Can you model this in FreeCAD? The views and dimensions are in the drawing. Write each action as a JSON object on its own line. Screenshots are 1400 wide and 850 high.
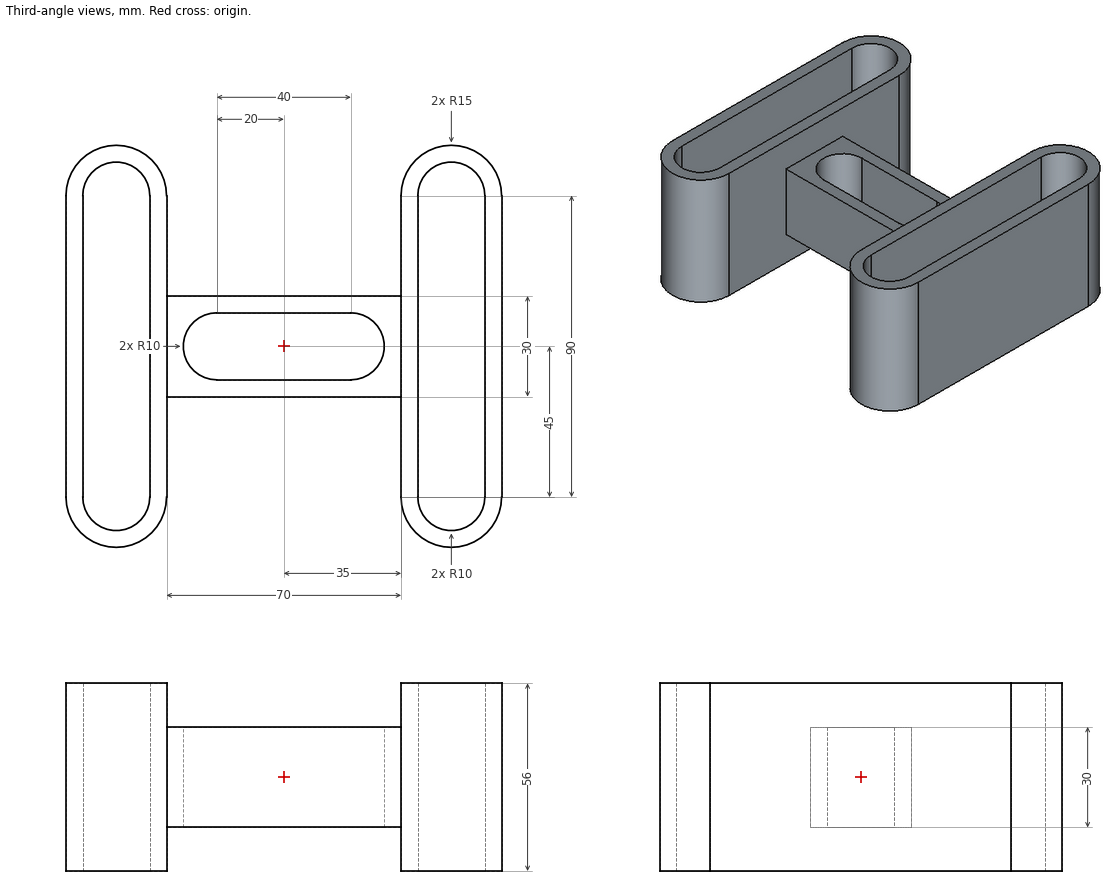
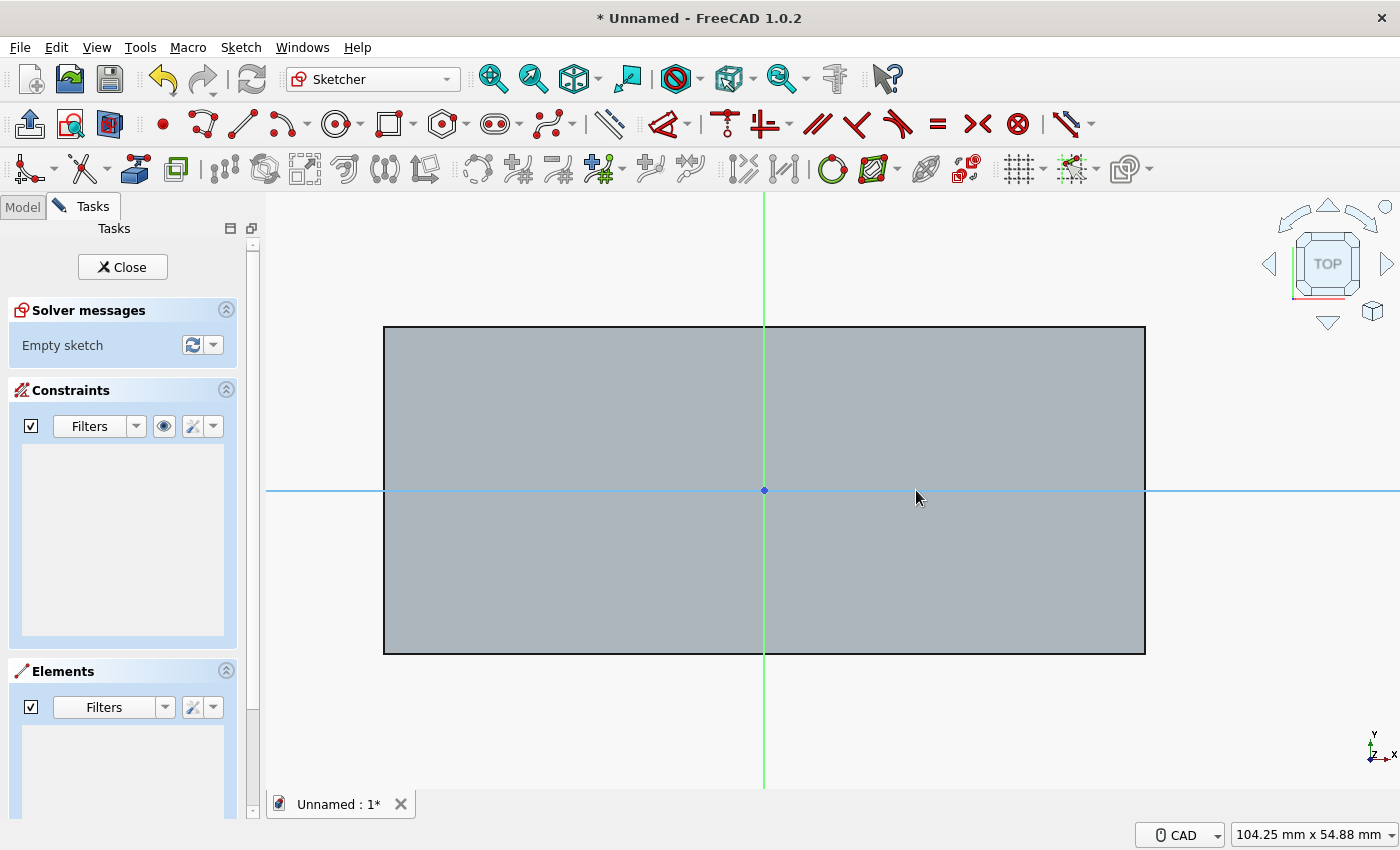
{"action": "left_click", "coordinate": [496, 124]}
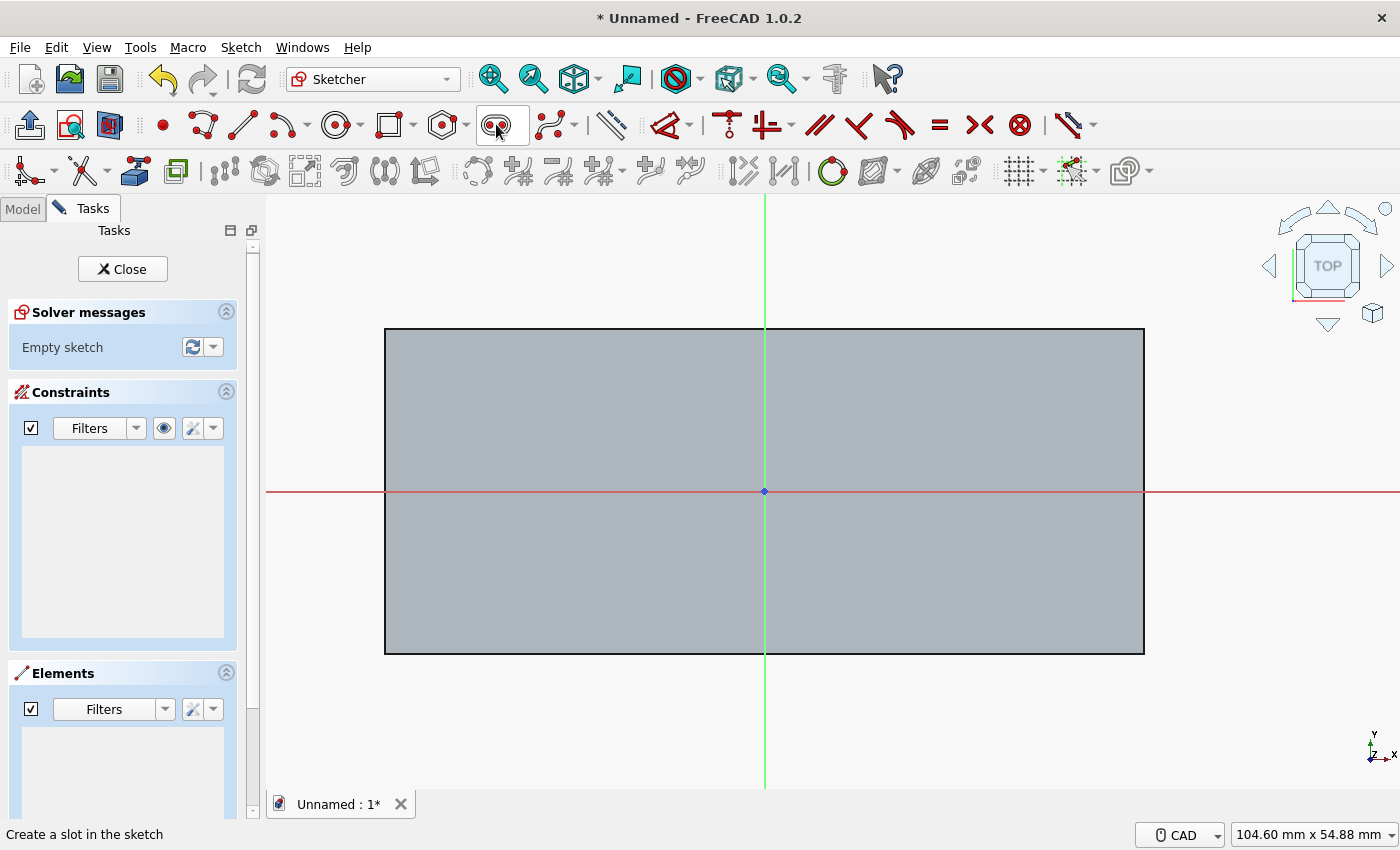
{"action": "left_click", "coordinate": [548, 492]}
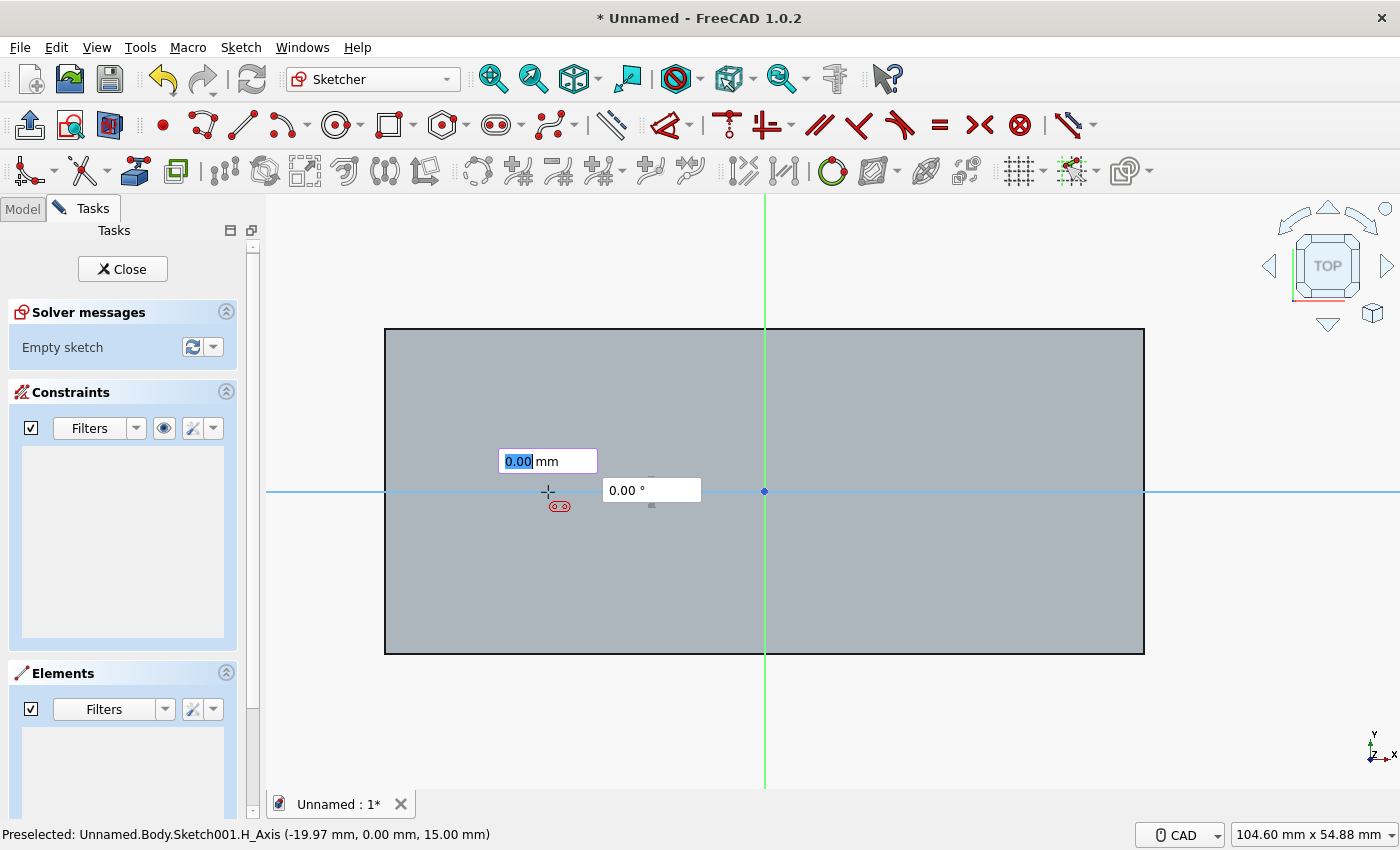
{"action": "left_click", "coordinate": [981, 482]}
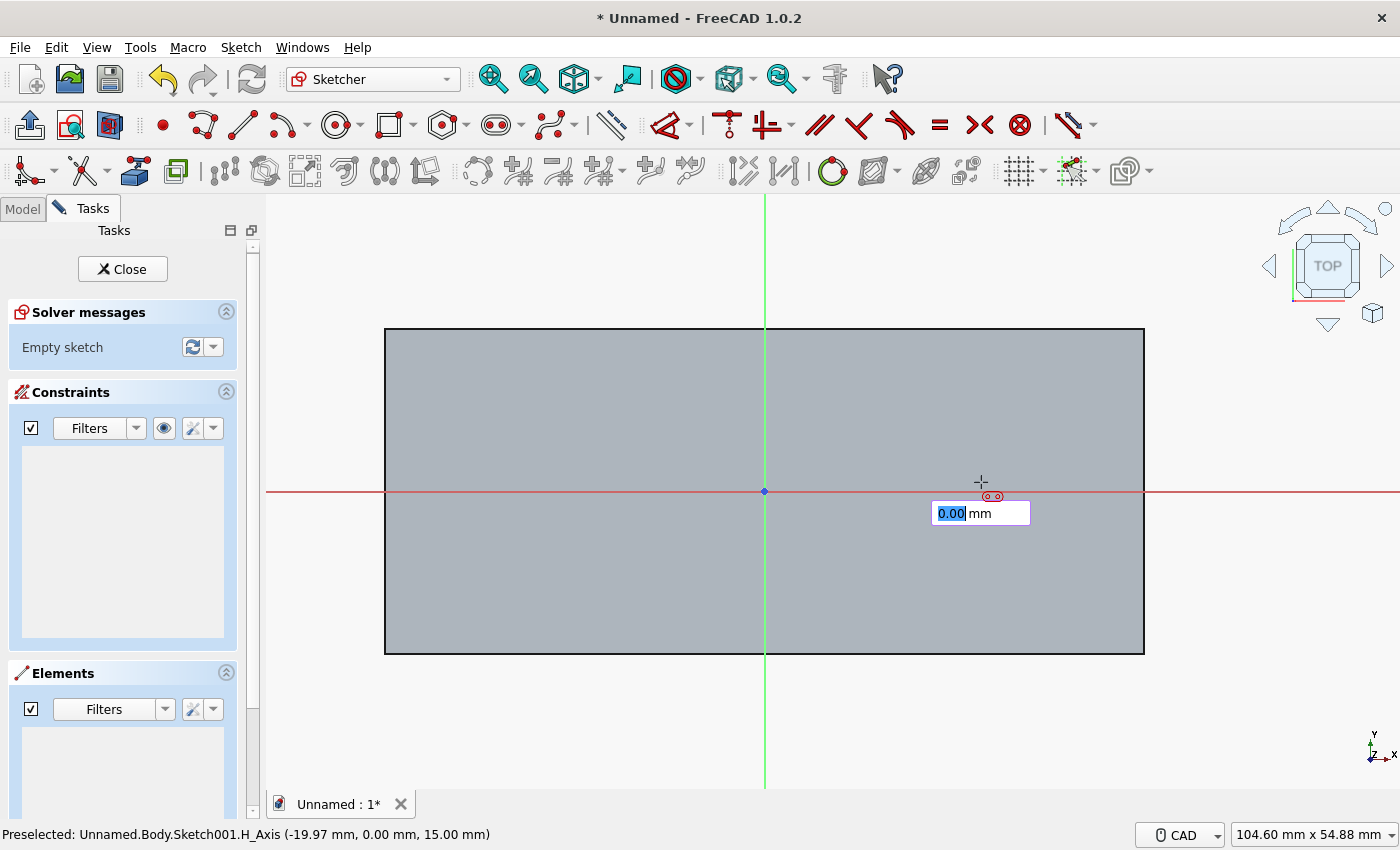
{"action": "left_click", "coordinate": [830, 383]}
{"action": "key", "text": "Escape"}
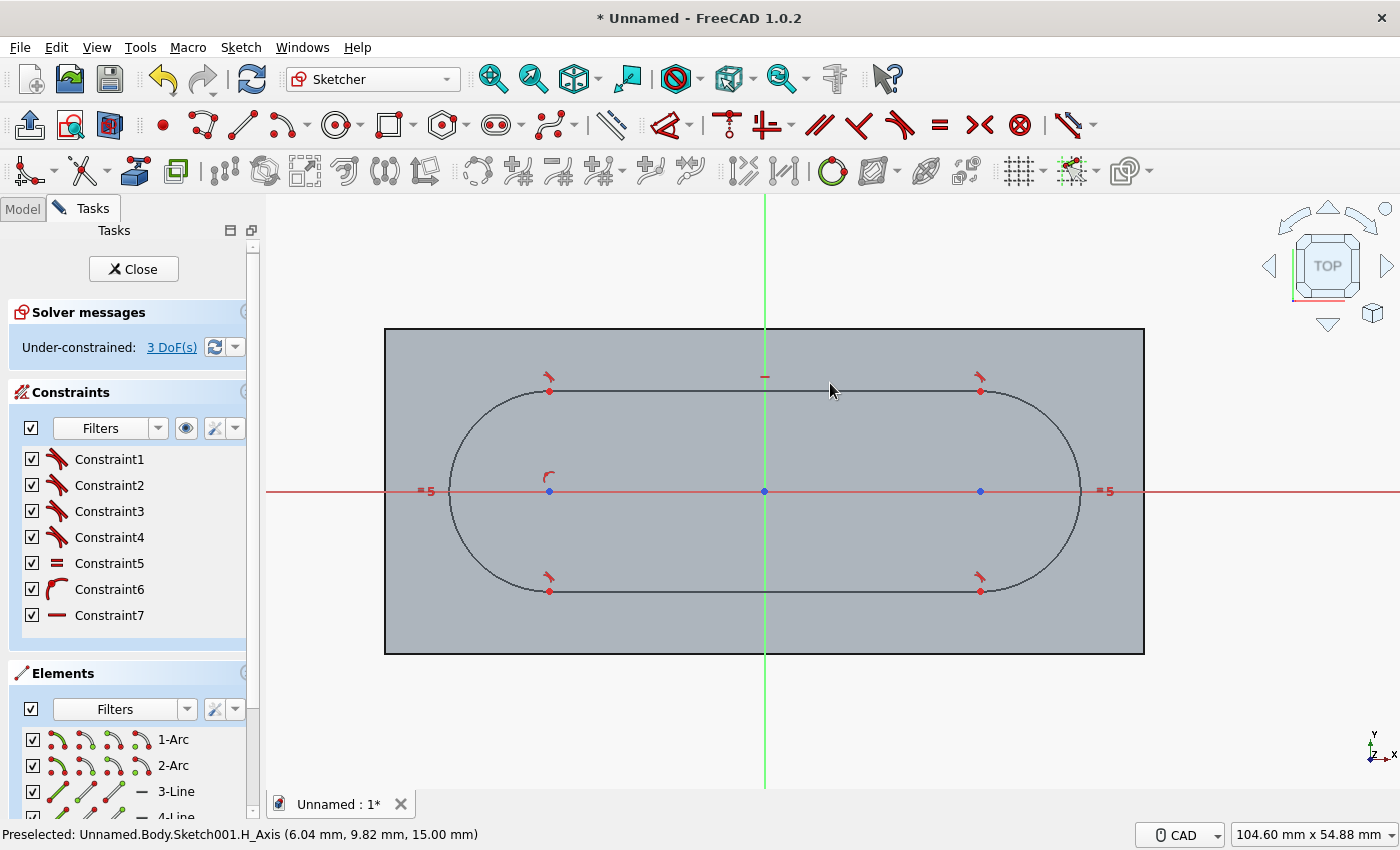
{"action": "left_click", "coordinate": [468, 433]}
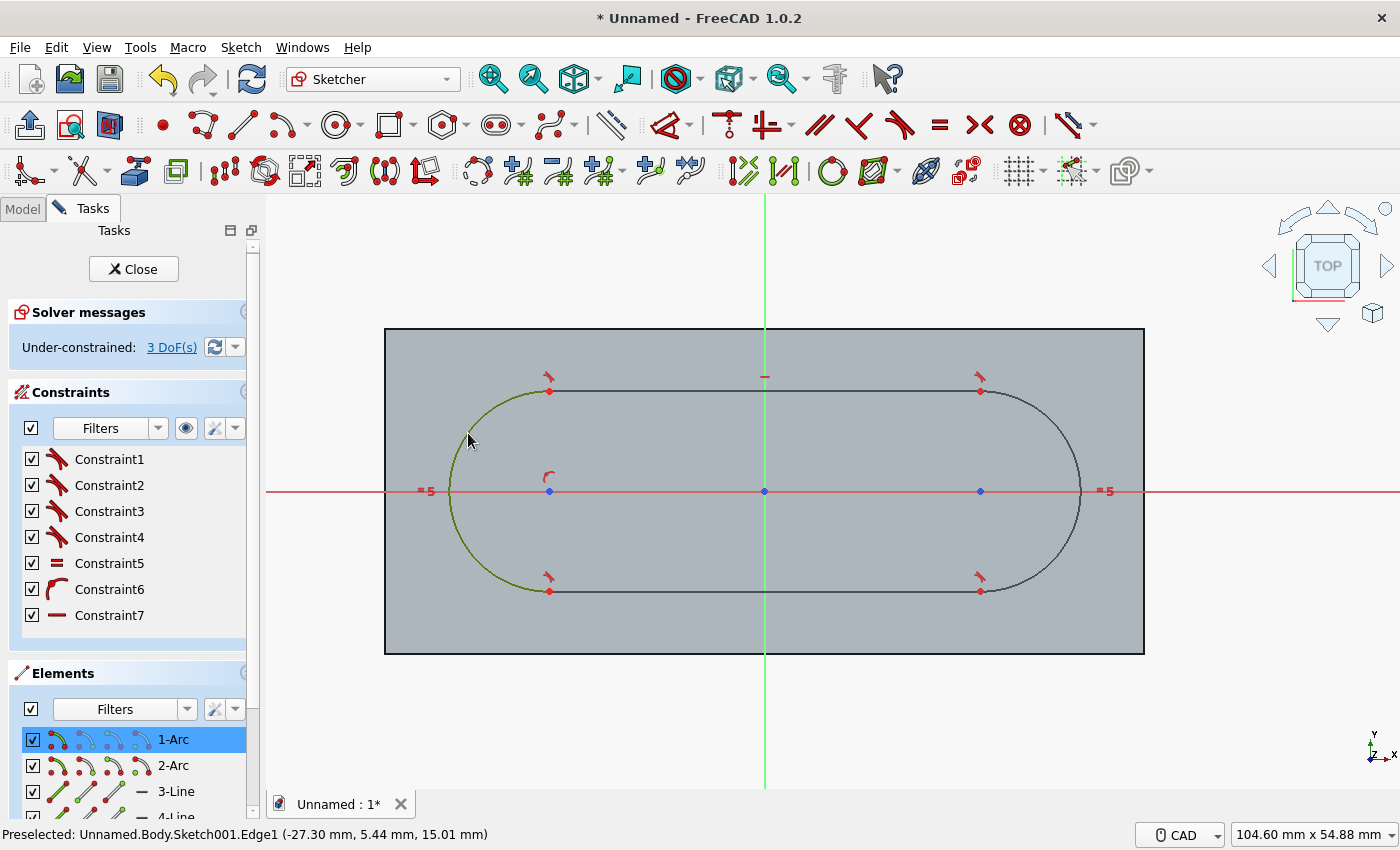
{"action": "key", "text": "k r"}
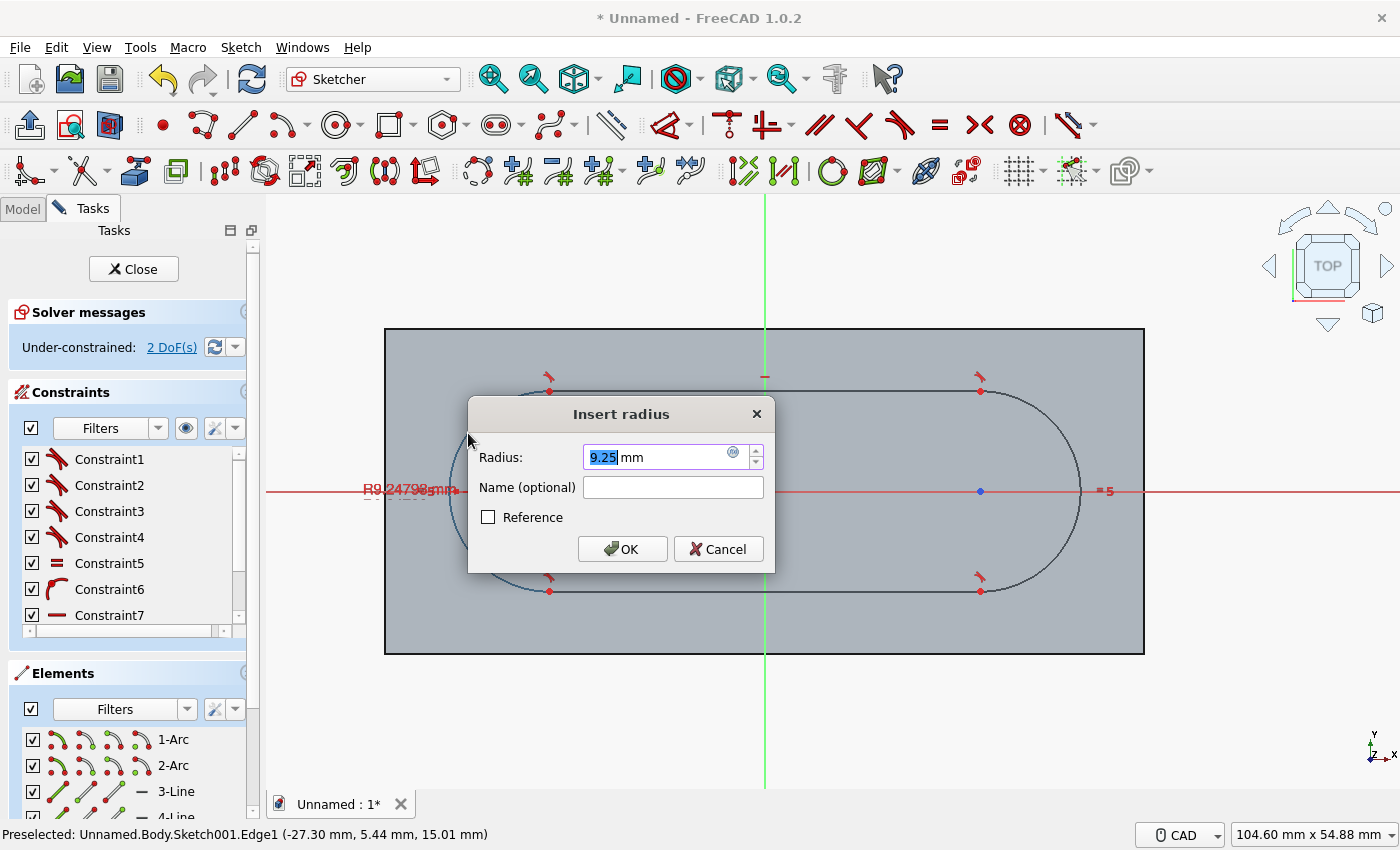
{"action": "type", "text": "10"}
{"action": "key", "text": "Return"}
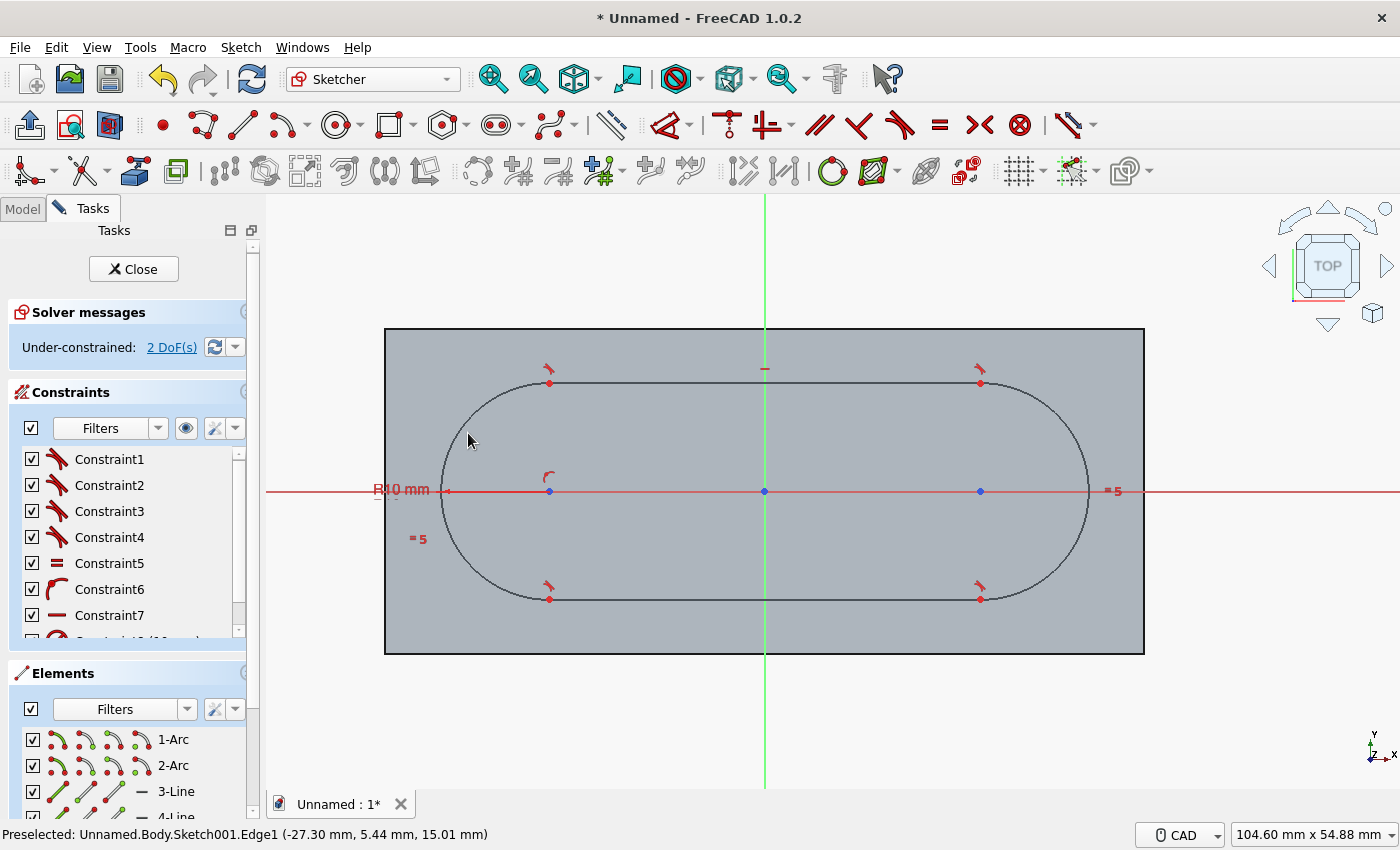
{"action": "left_click", "coordinate": [679, 383]}